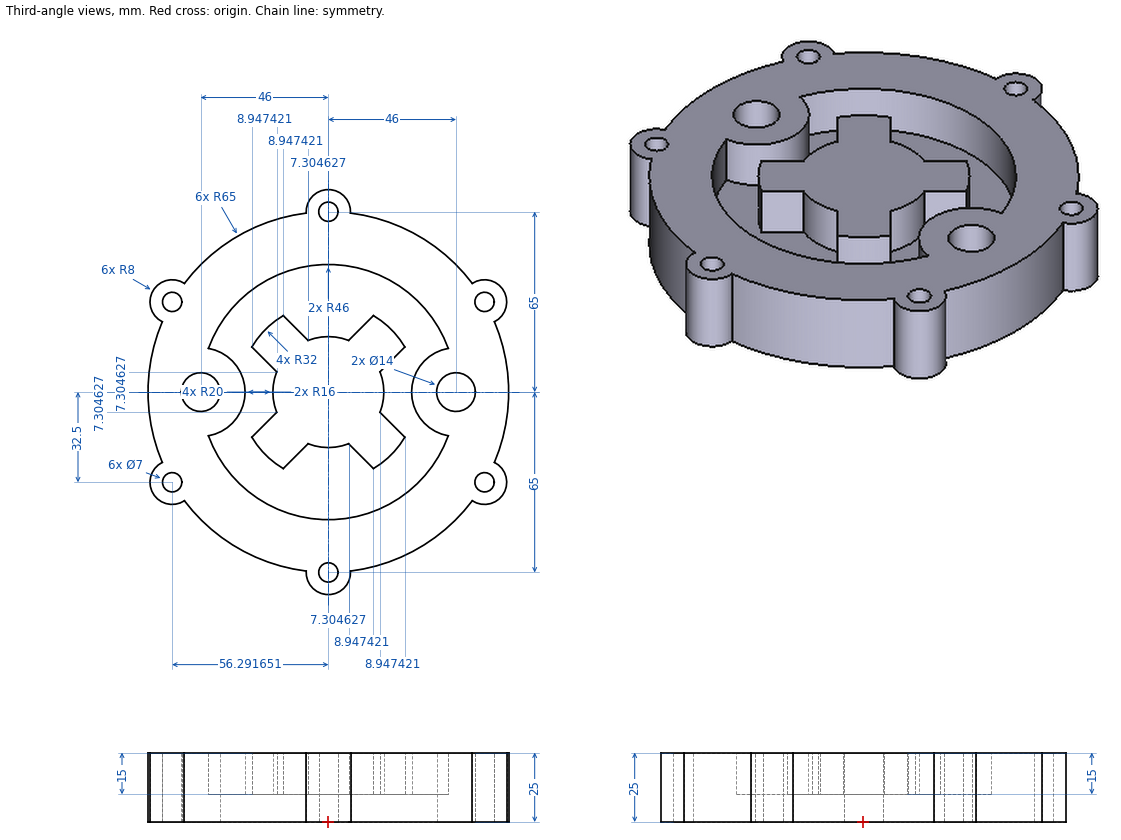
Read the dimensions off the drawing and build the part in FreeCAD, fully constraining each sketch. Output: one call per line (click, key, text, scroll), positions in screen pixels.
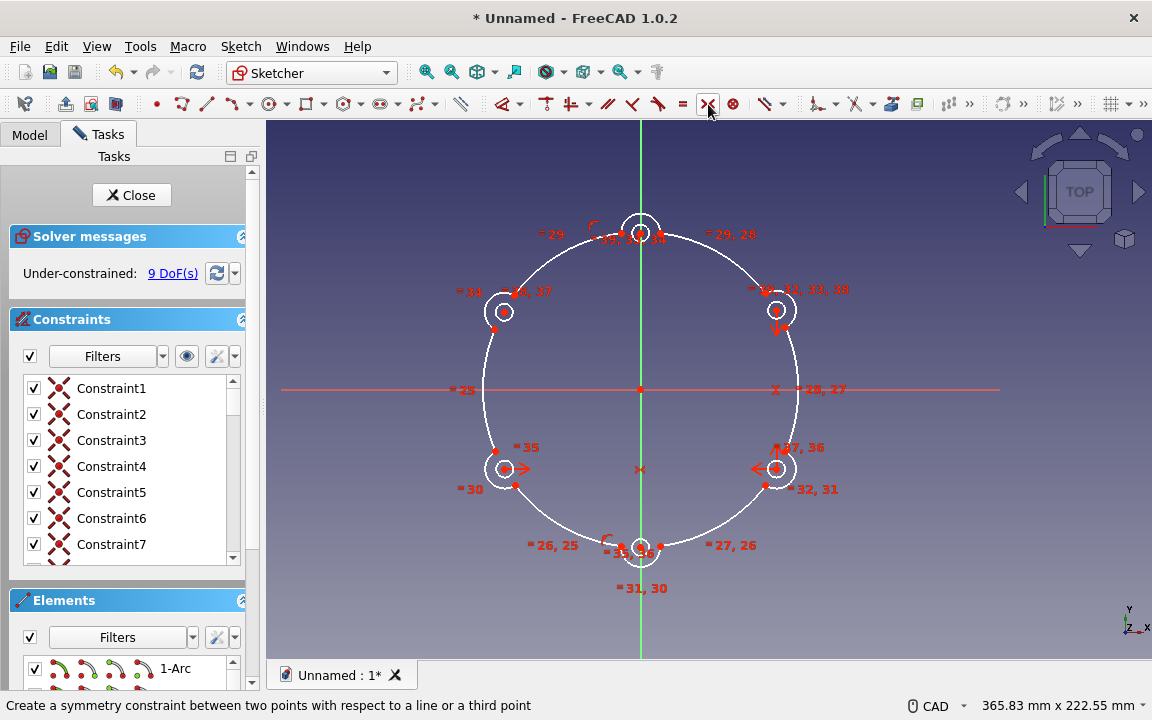
click(505, 469)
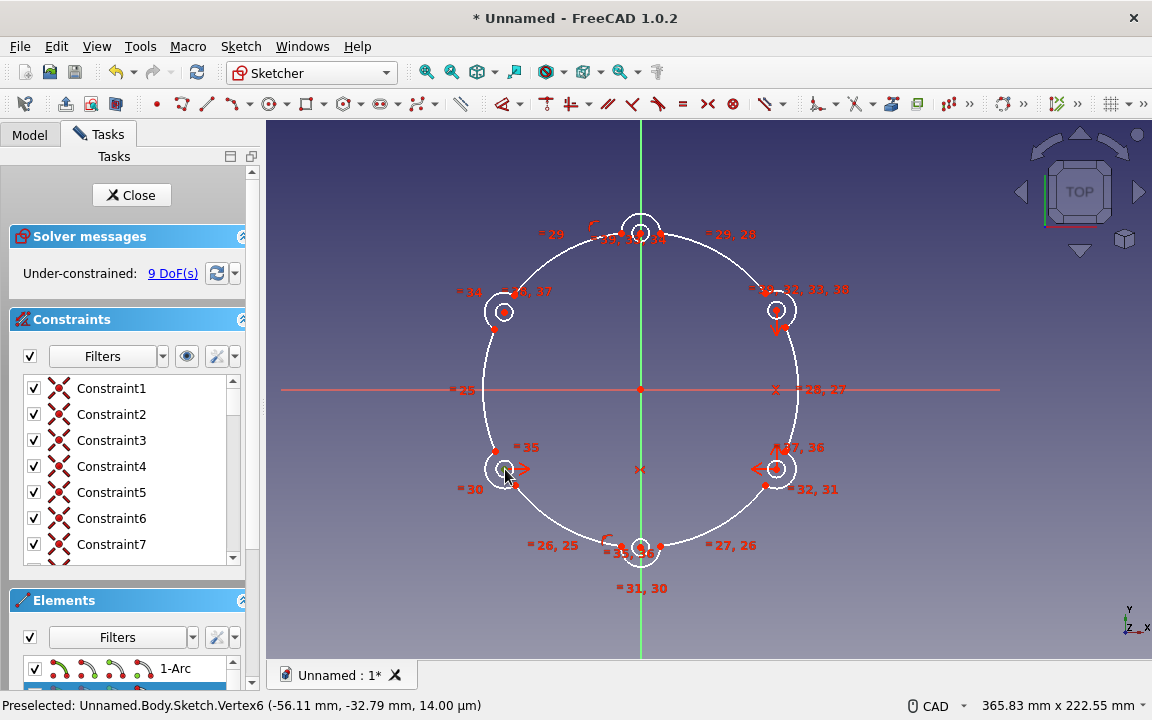
click(504, 312)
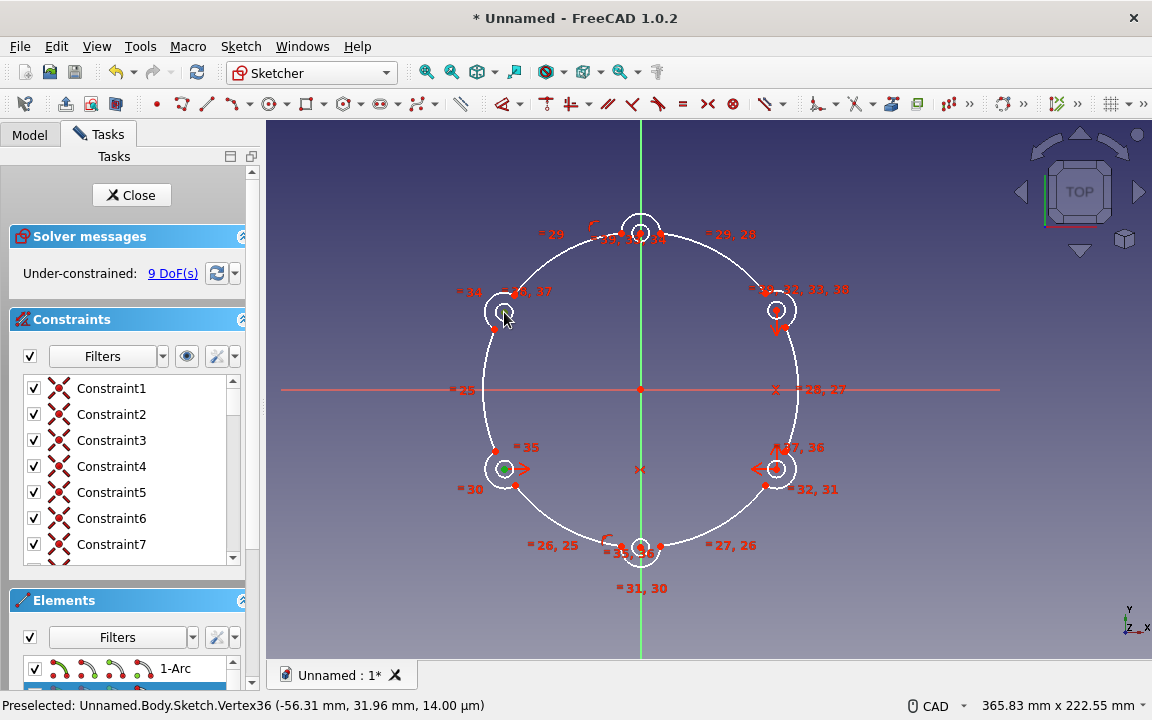
click(344, 390)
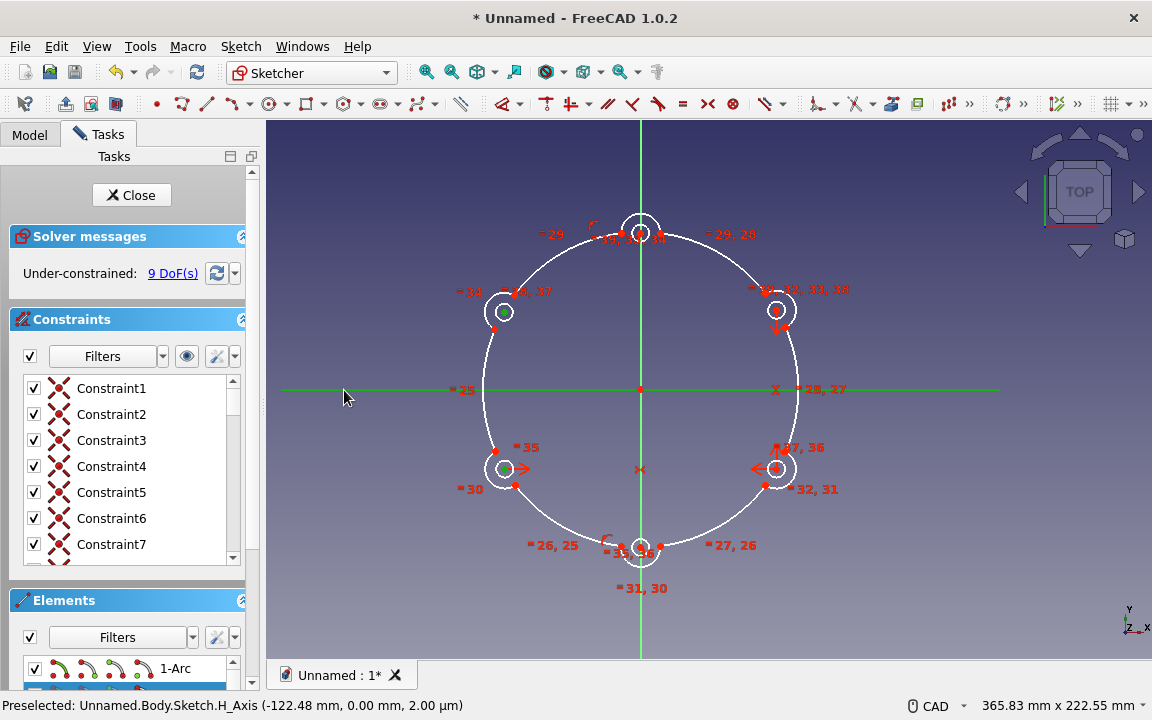
click(708, 104)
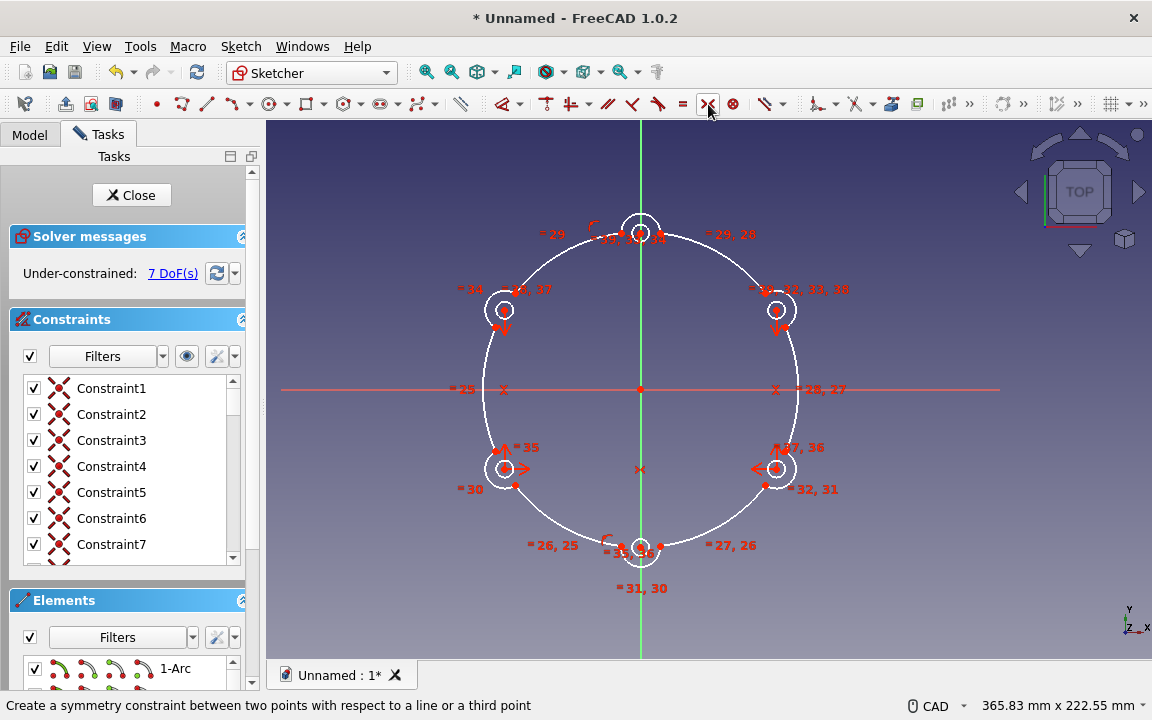
click(485, 364)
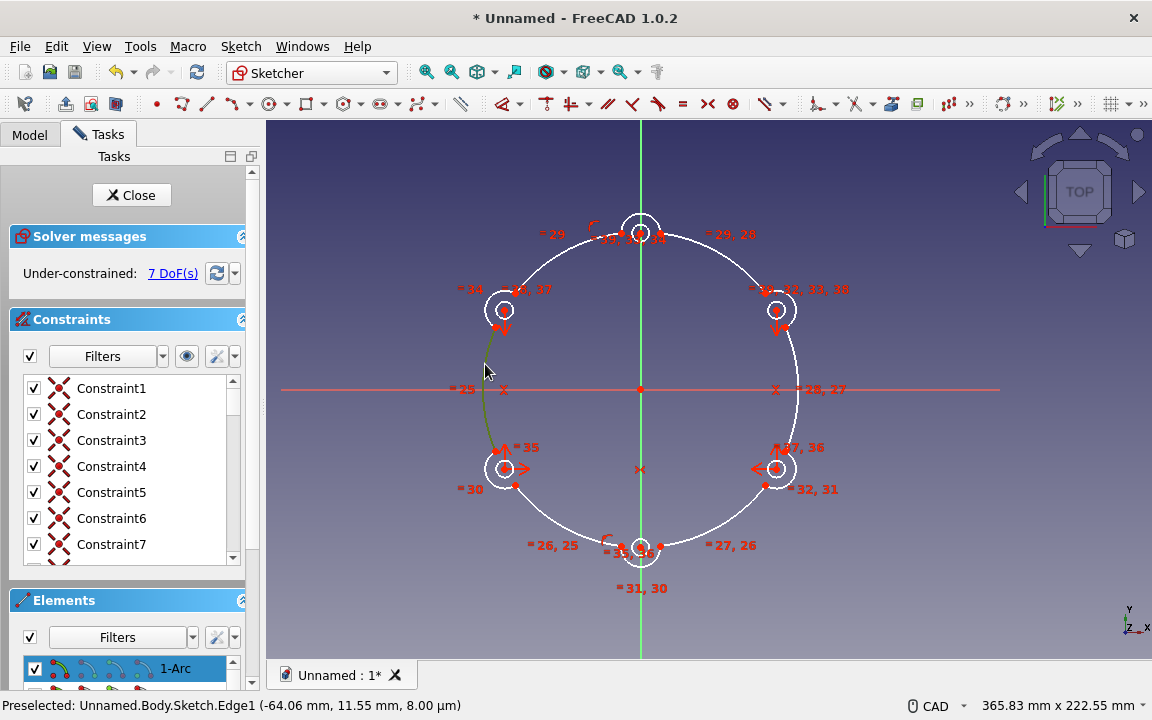
click(520, 104)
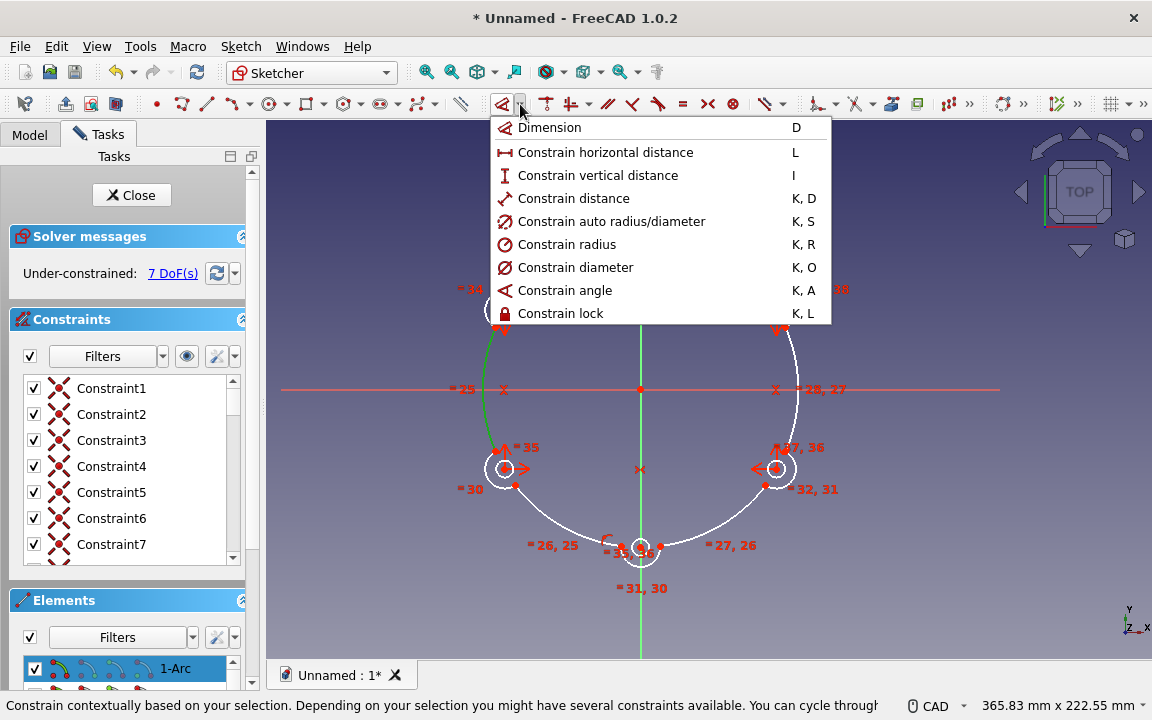
click(661, 244)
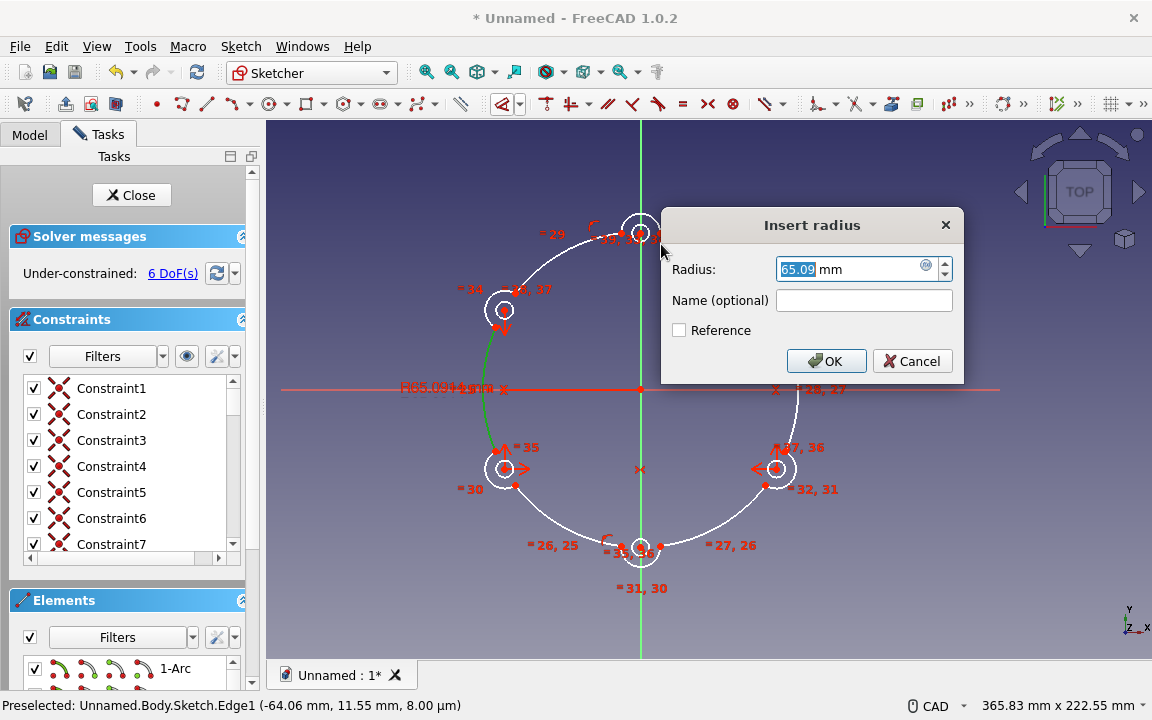
text(65)
key(Return)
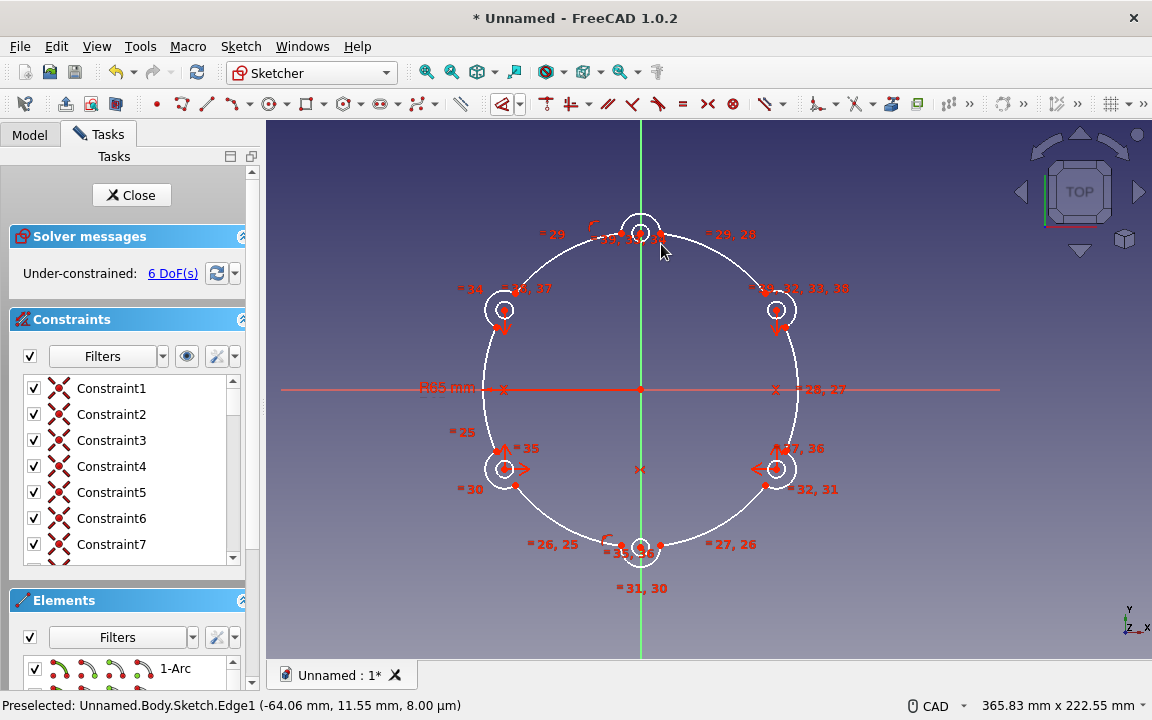
scroll(485, 467, up, 4)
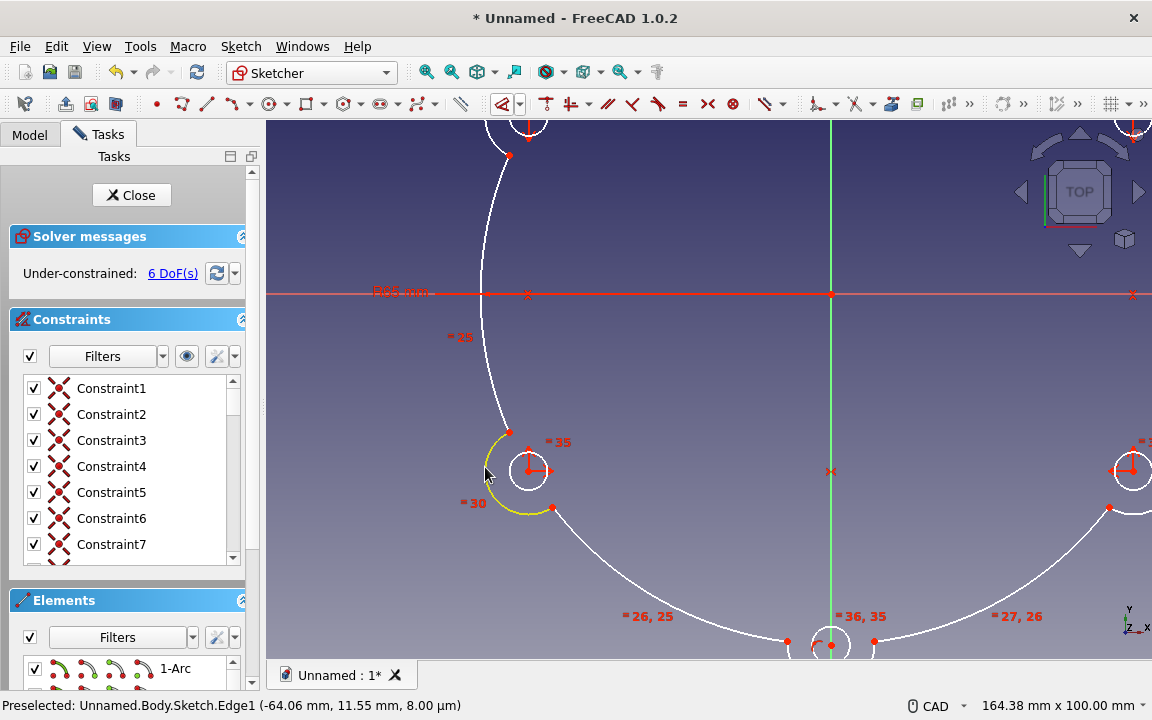
click(486, 466)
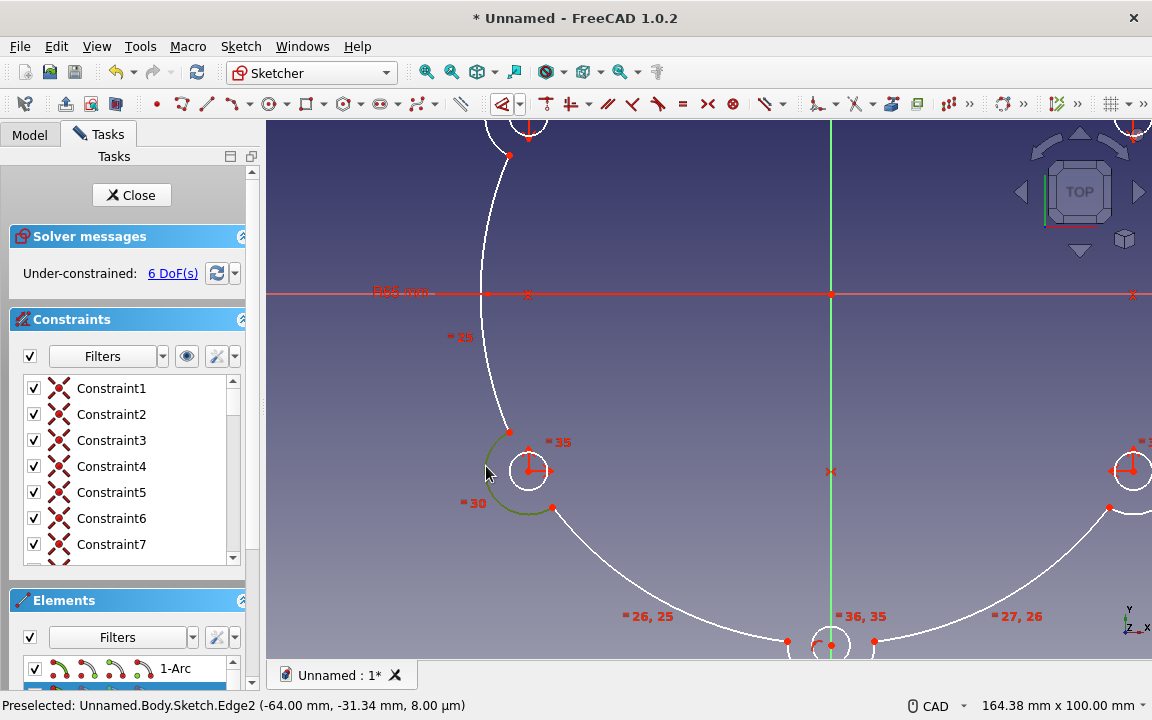
click(520, 104)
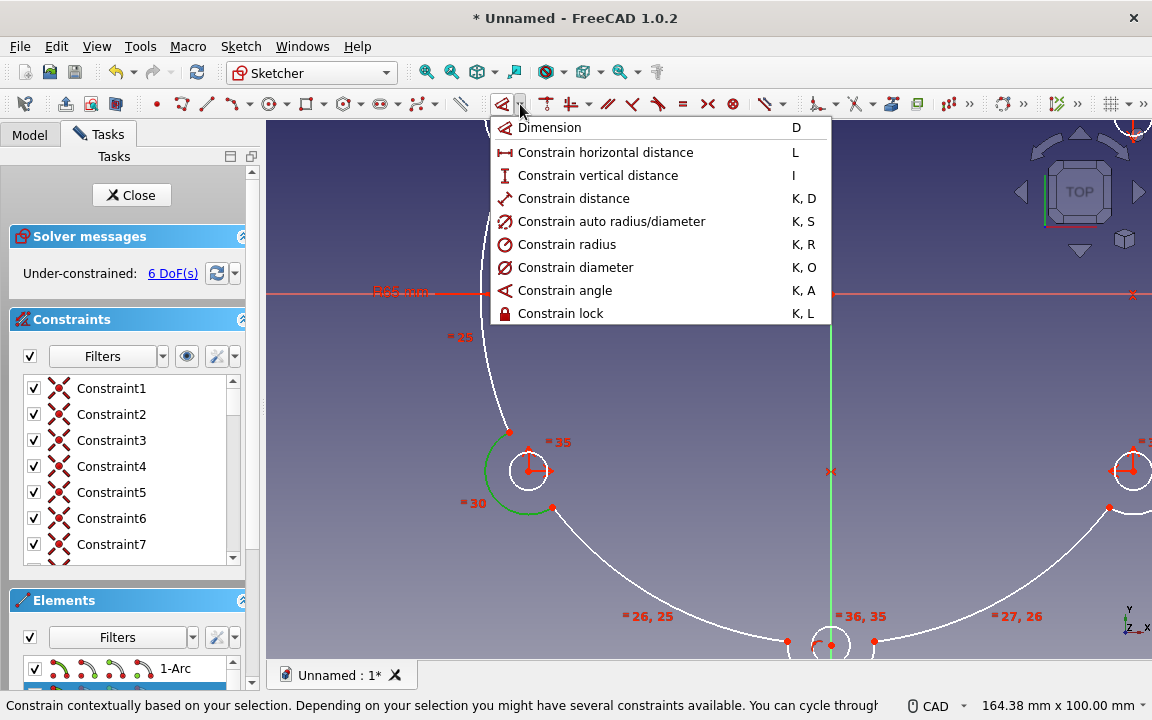
click(661, 244)